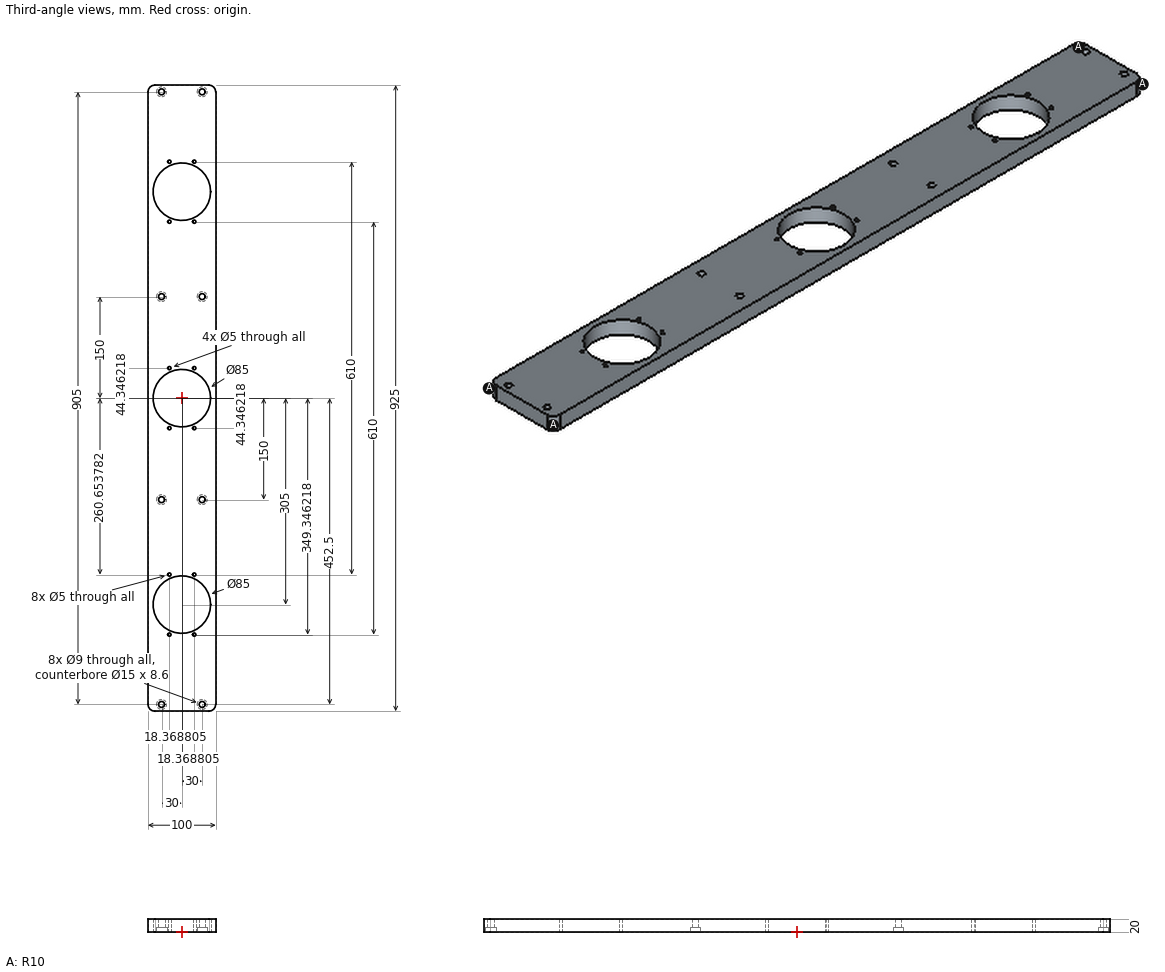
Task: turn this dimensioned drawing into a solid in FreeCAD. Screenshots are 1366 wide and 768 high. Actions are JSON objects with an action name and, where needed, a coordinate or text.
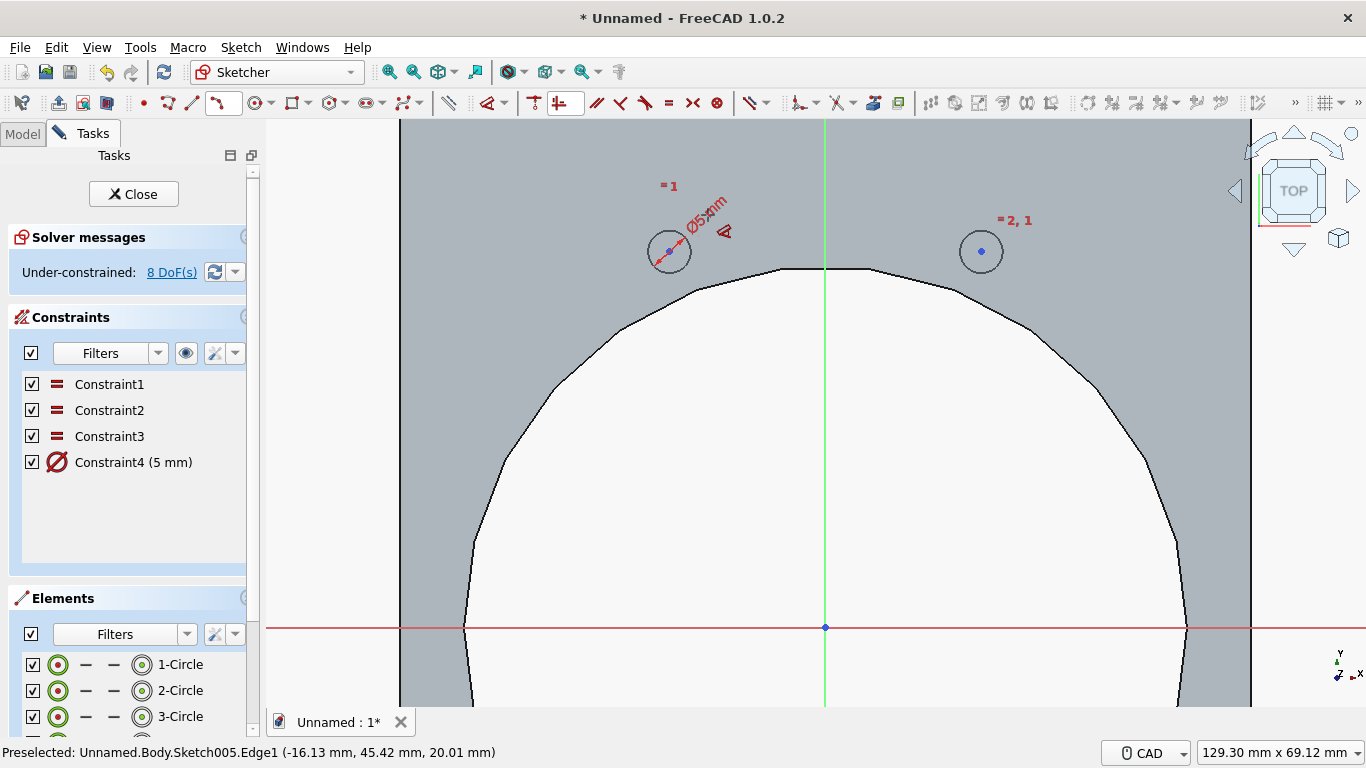
{"action": "left_click", "coordinate": [669, 252]}
{"action": "left_click", "coordinate": [783, 218]}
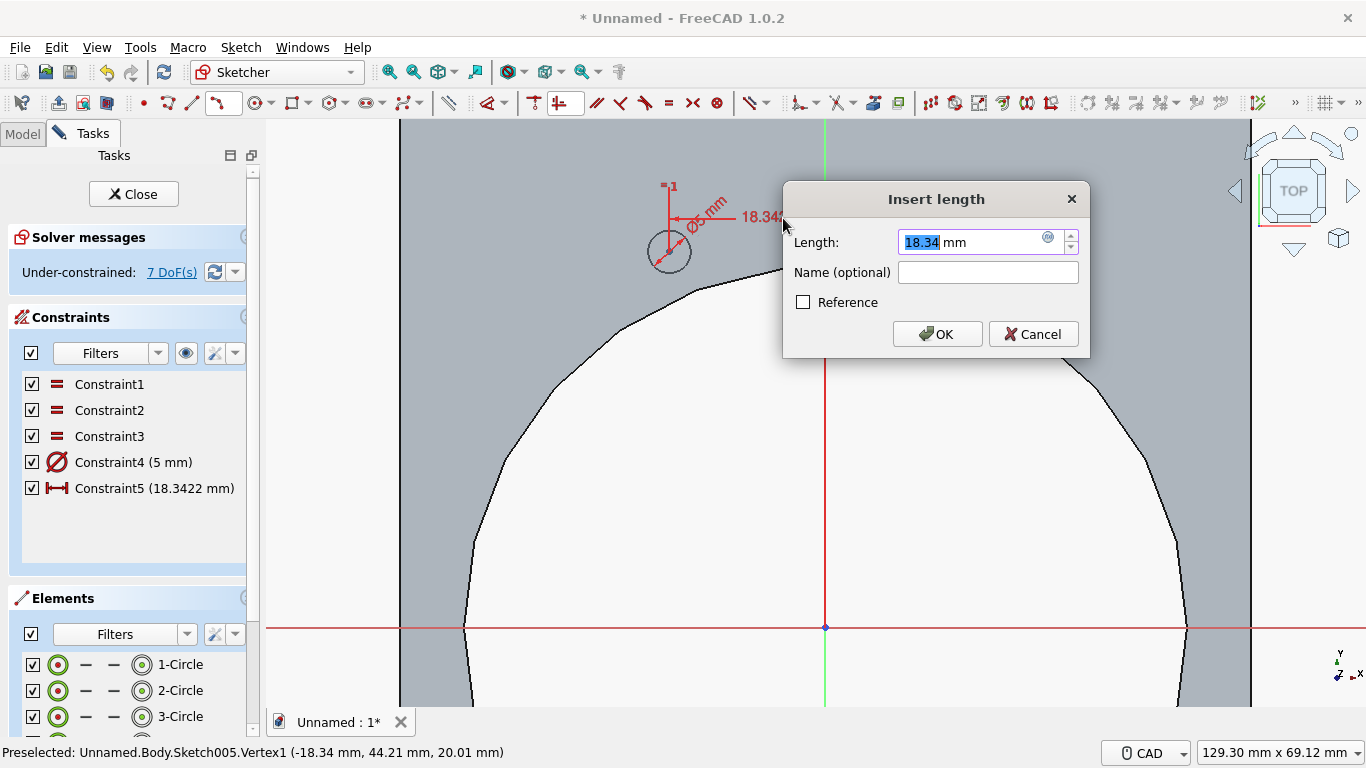
{"action": "type", "text": "18.368805"}
{"action": "key", "text": "Return"}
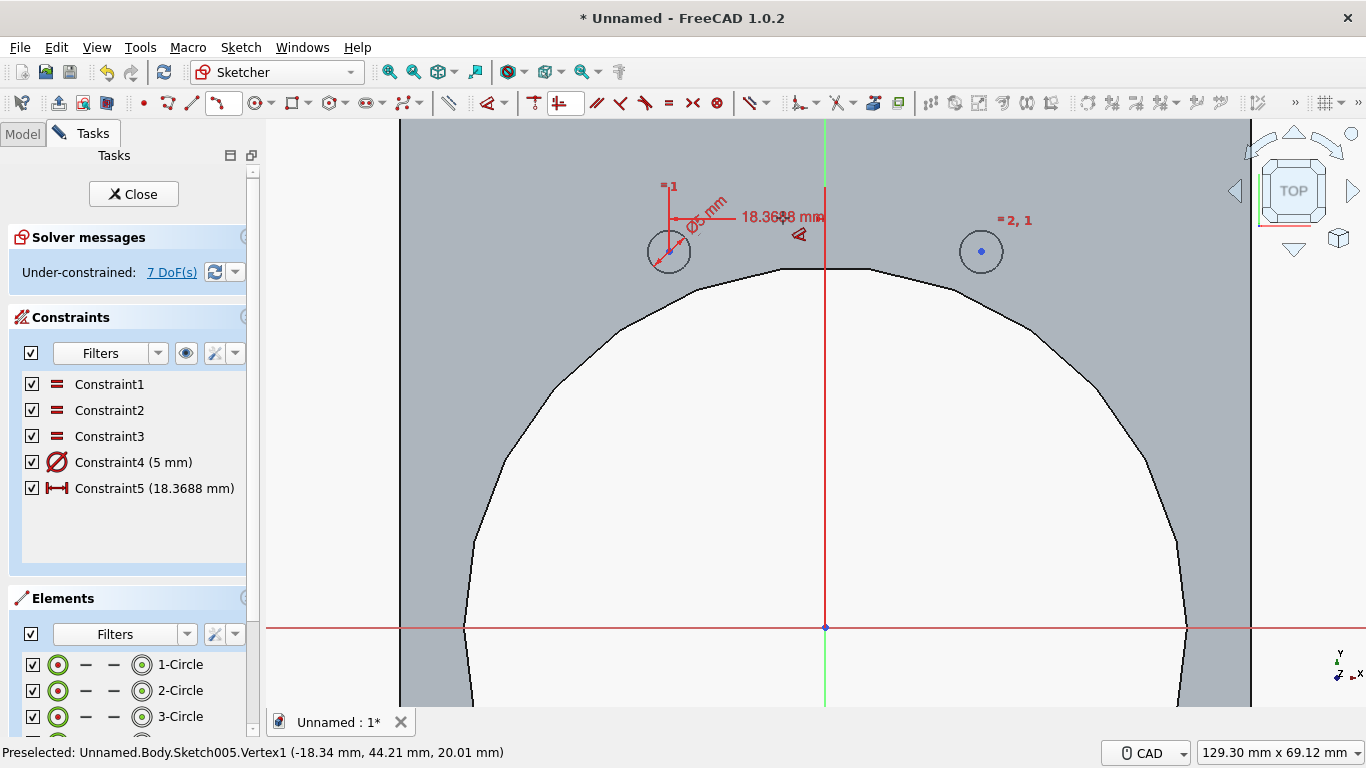
{"action": "left_click", "coordinate": [669, 252]}
{"action": "left_click", "coordinate": [635, 440]}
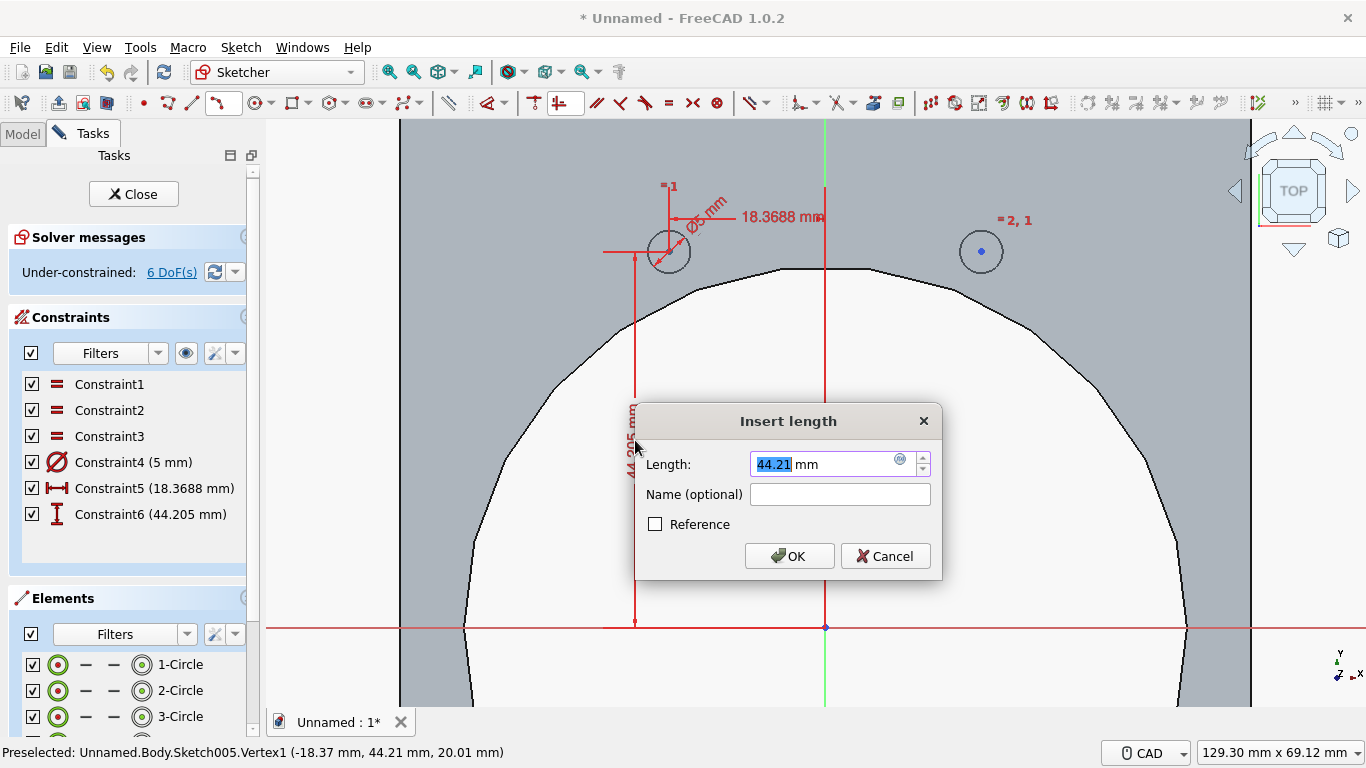
{"action": "type", "text": "44.346218"}
{"action": "key", "text": "Return"}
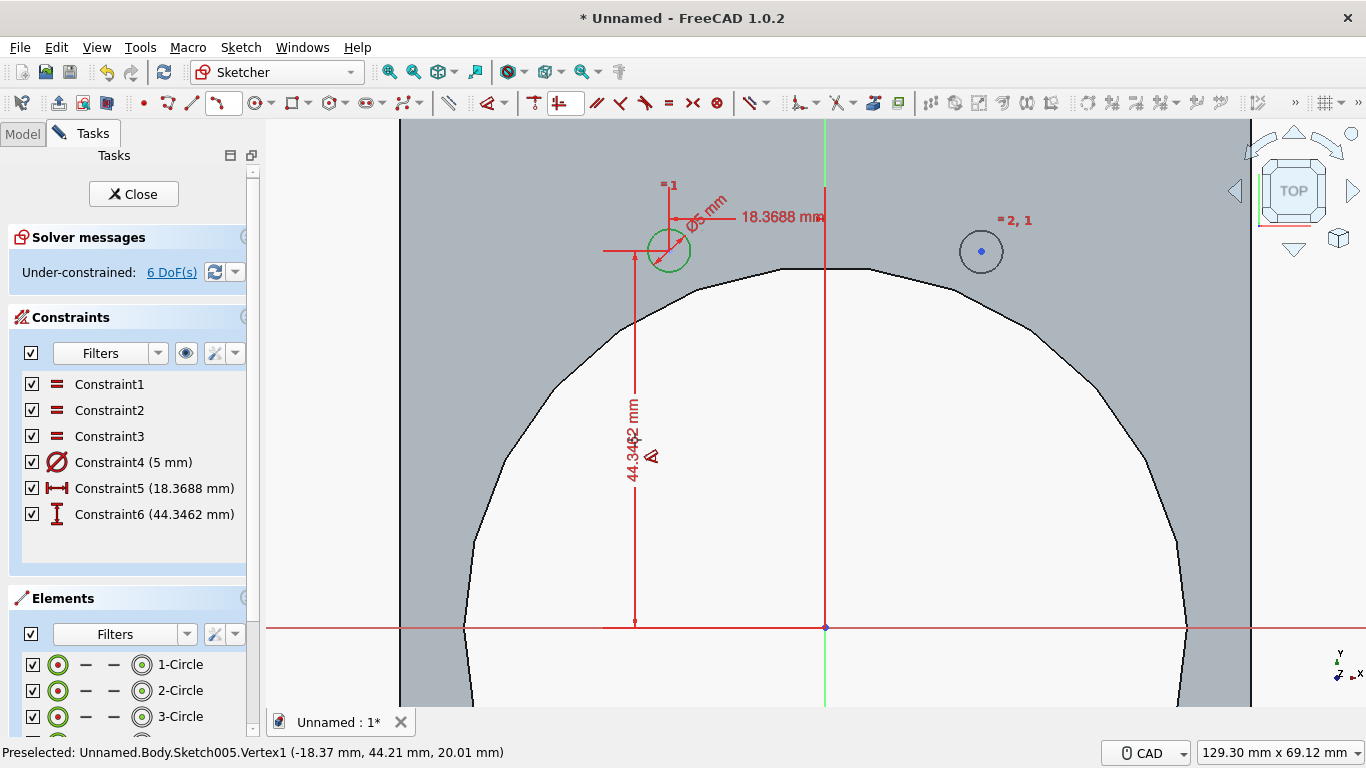
{"action": "left_click", "coordinate": [981, 252]}
{"action": "left_click", "coordinate": [903, 218]}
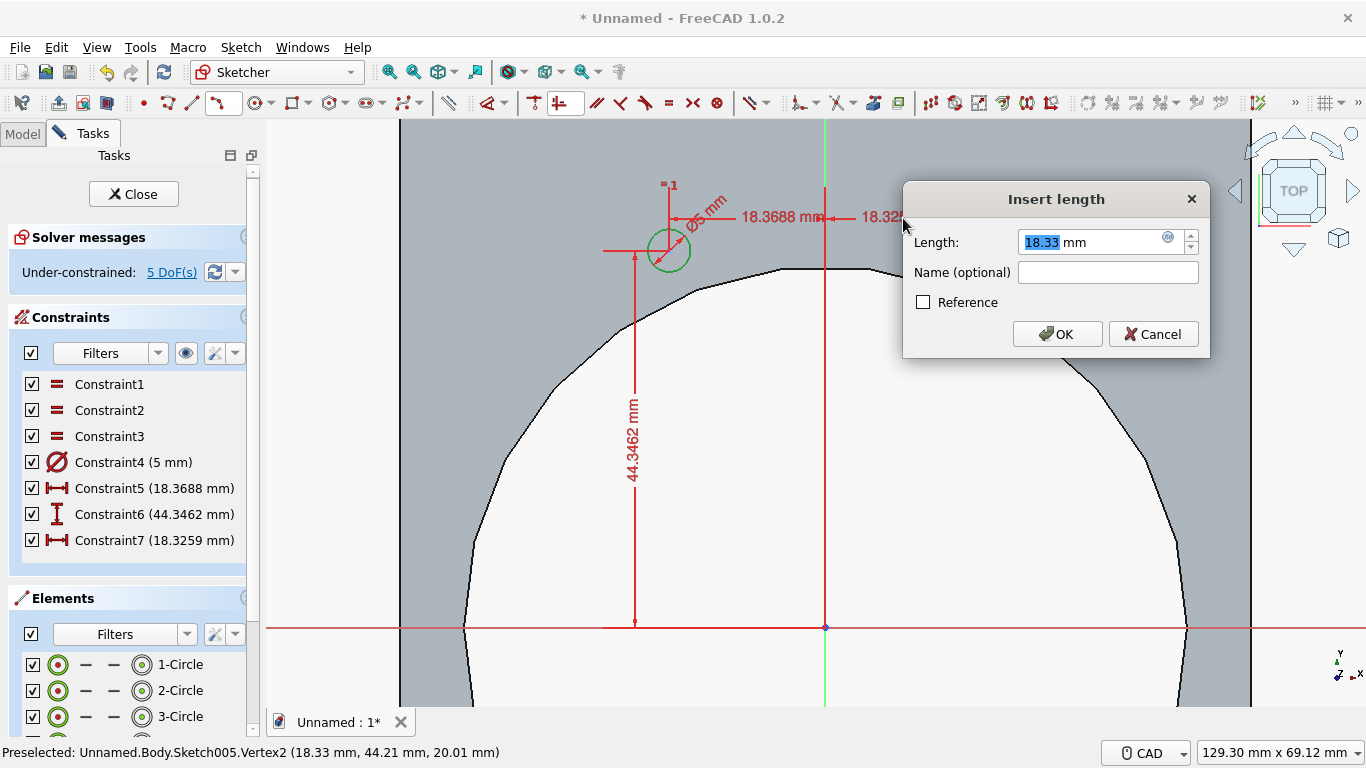
{"action": "type", "text": "18.368805"}
{"action": "key", "text": "Return"}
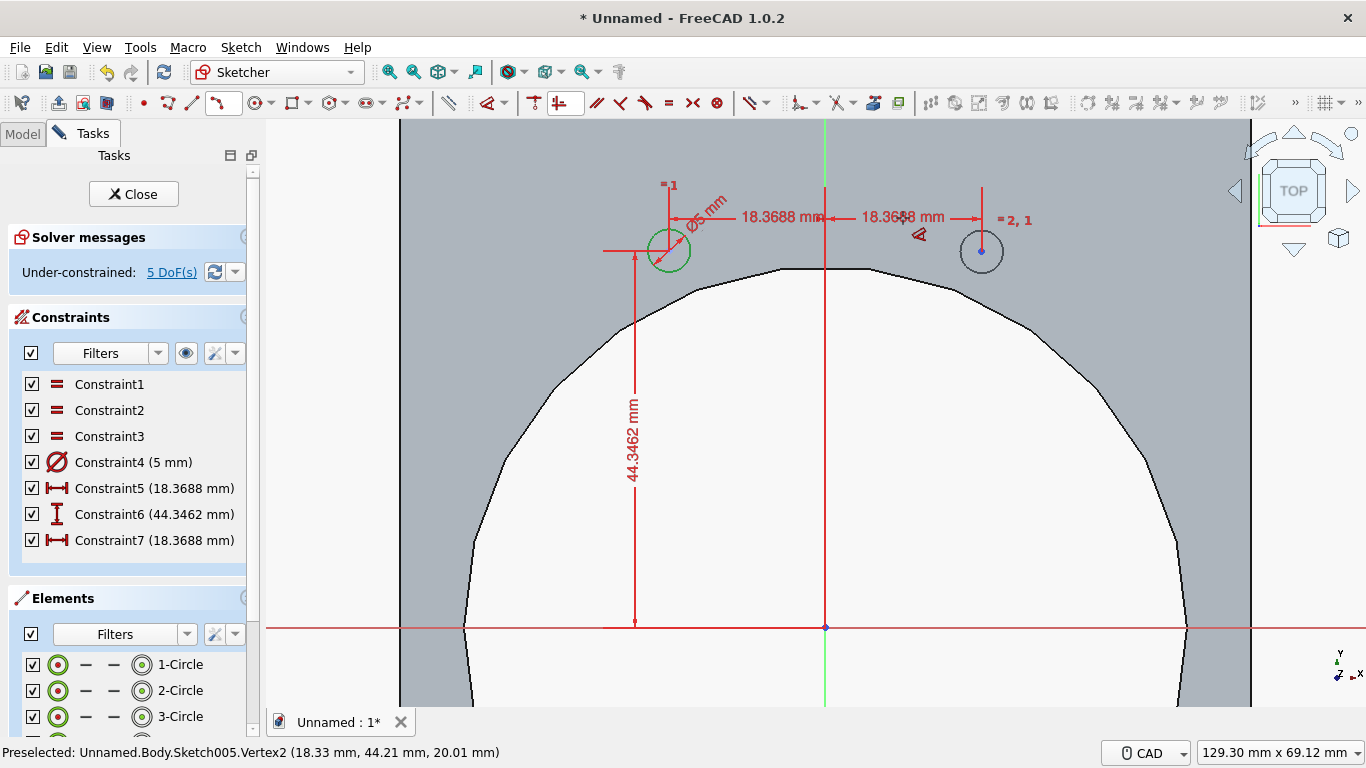
{"action": "left_click", "coordinate": [982, 252]}
{"action": "left_click", "coordinate": [1016, 440]}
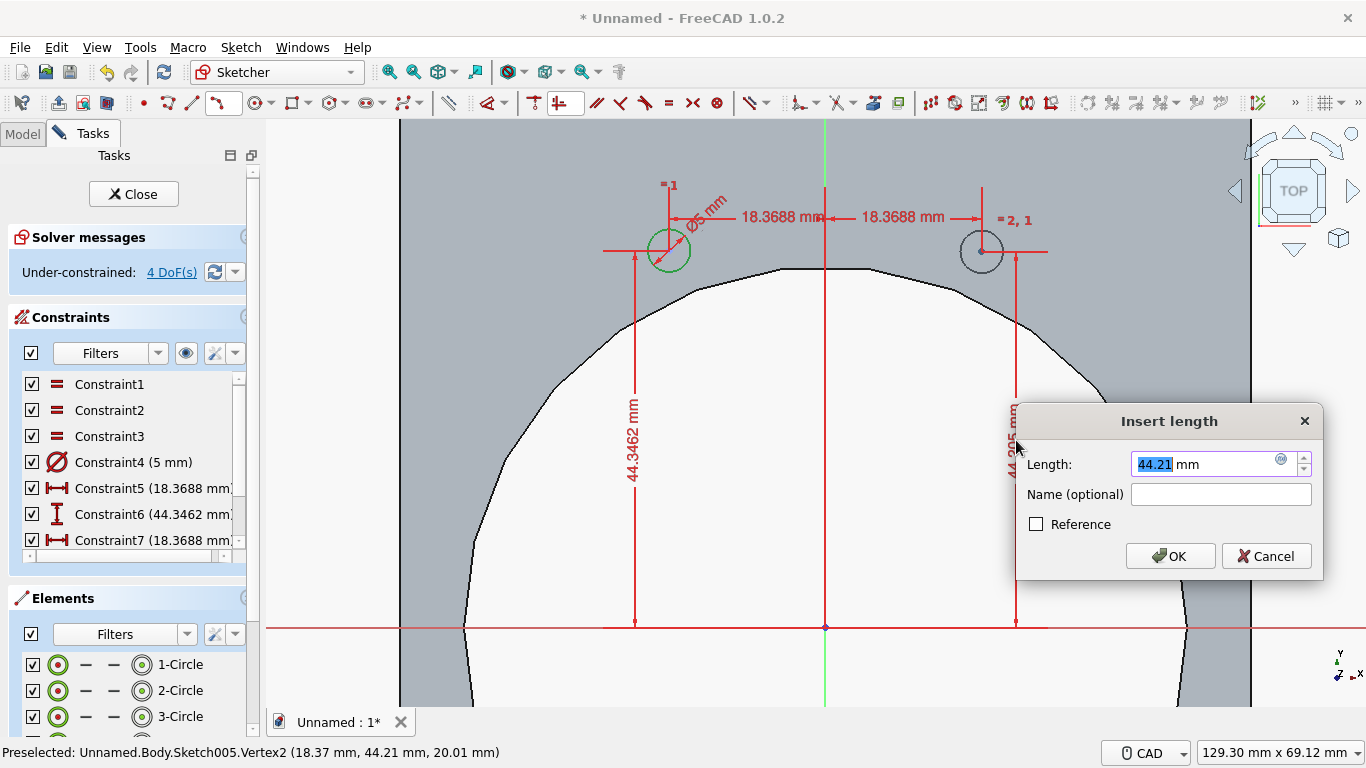
{"action": "type", "text": "44.346218"}
{"action": "key", "text": "Return"}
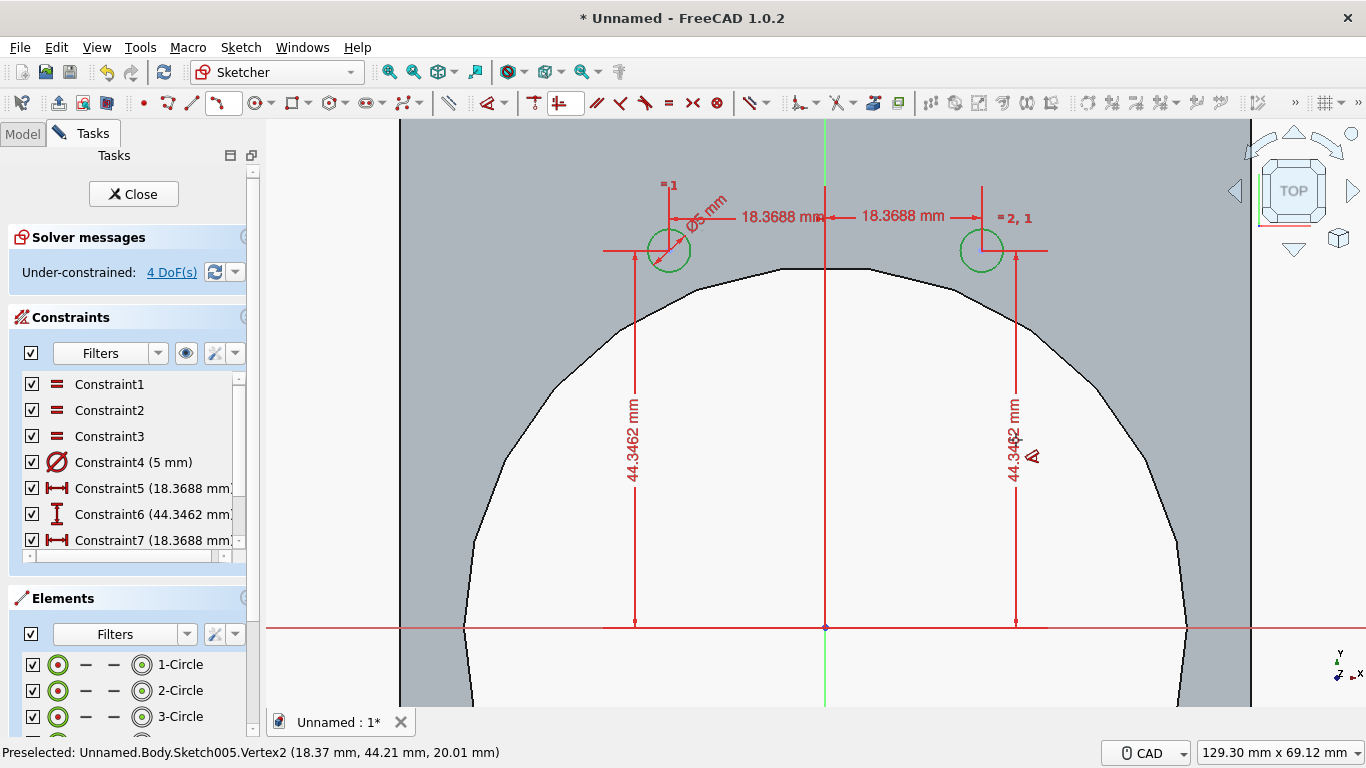
{"action": "scroll", "coordinate": [684, 238], "scroll_direction": "down", "scroll_amount": 4}